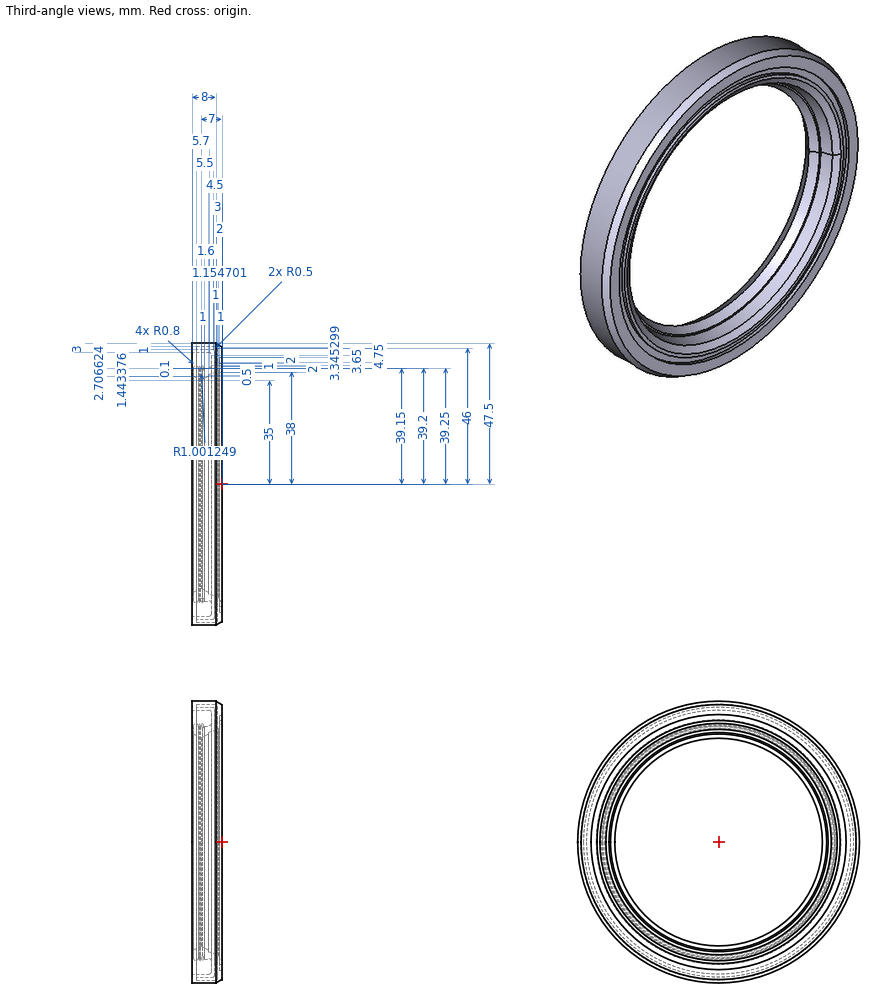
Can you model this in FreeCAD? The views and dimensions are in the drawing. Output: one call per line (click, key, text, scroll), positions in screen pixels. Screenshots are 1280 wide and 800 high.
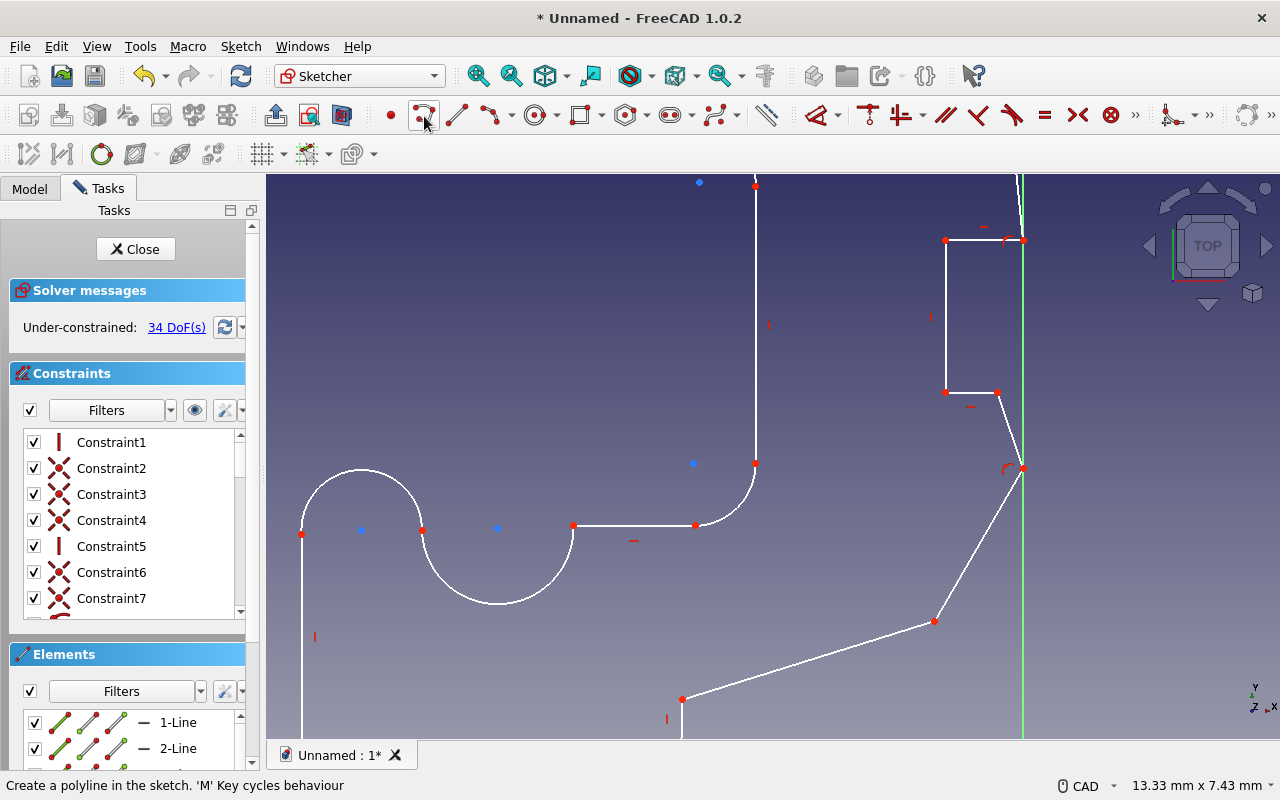
scroll(740, 507, down, 5)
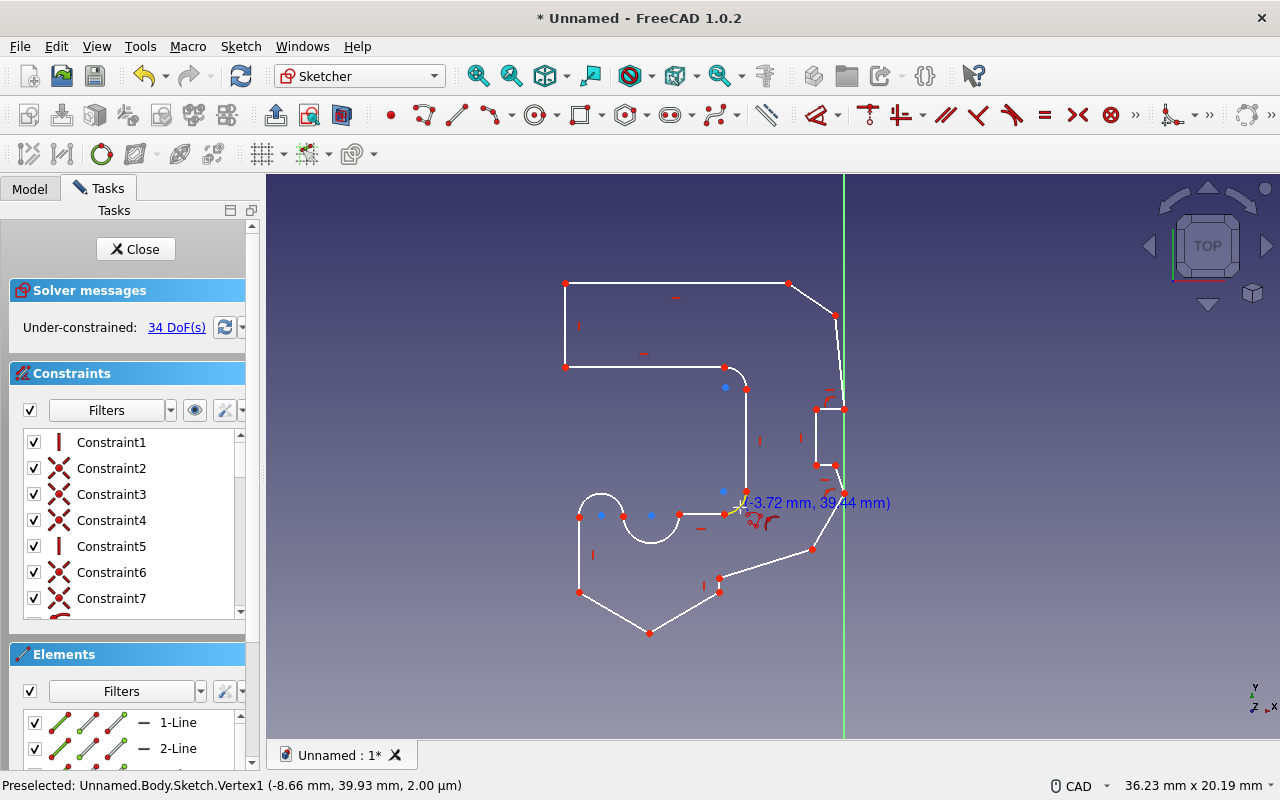
click(760, 338)
click(607, 338)
click(607, 310)
click(788, 310)
right_click(788, 310)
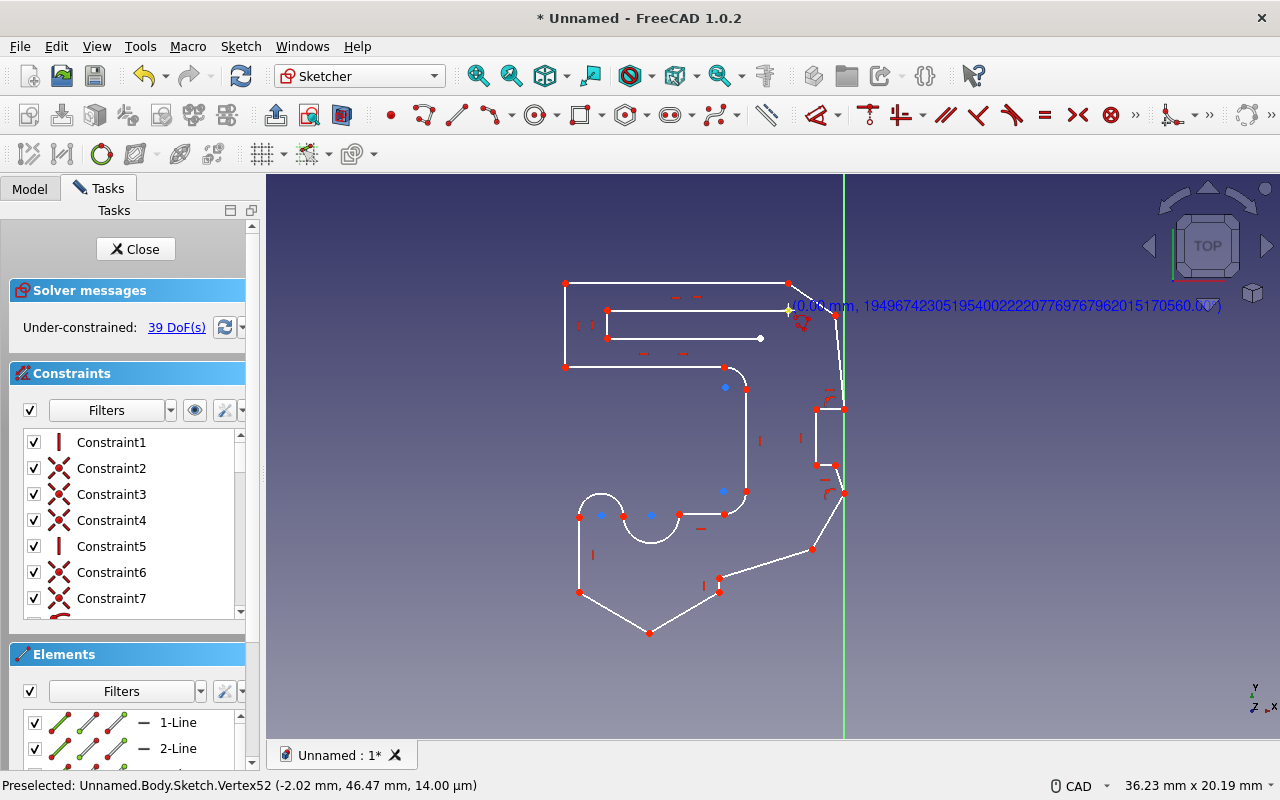
click(802, 324)
click(802, 457)
click(774, 457)
click(774, 352)
right_click(774, 352)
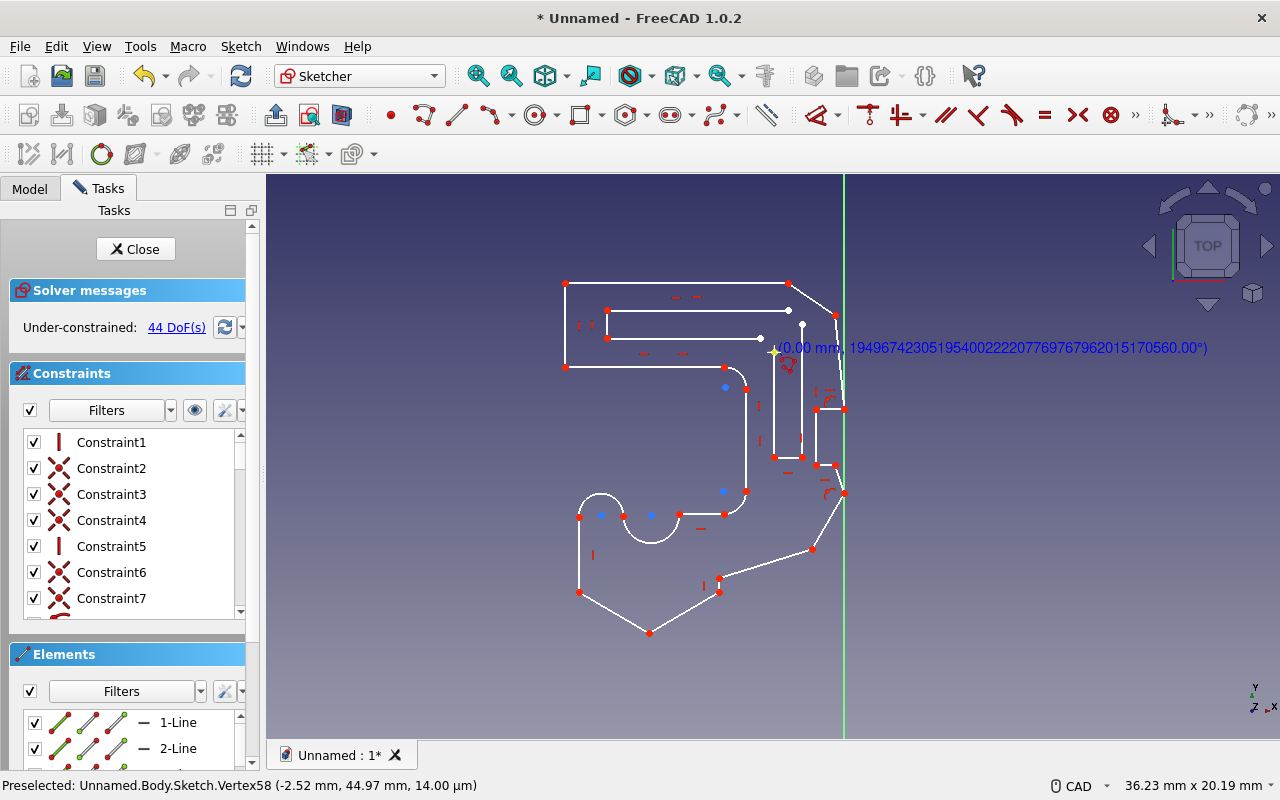
click(490, 116)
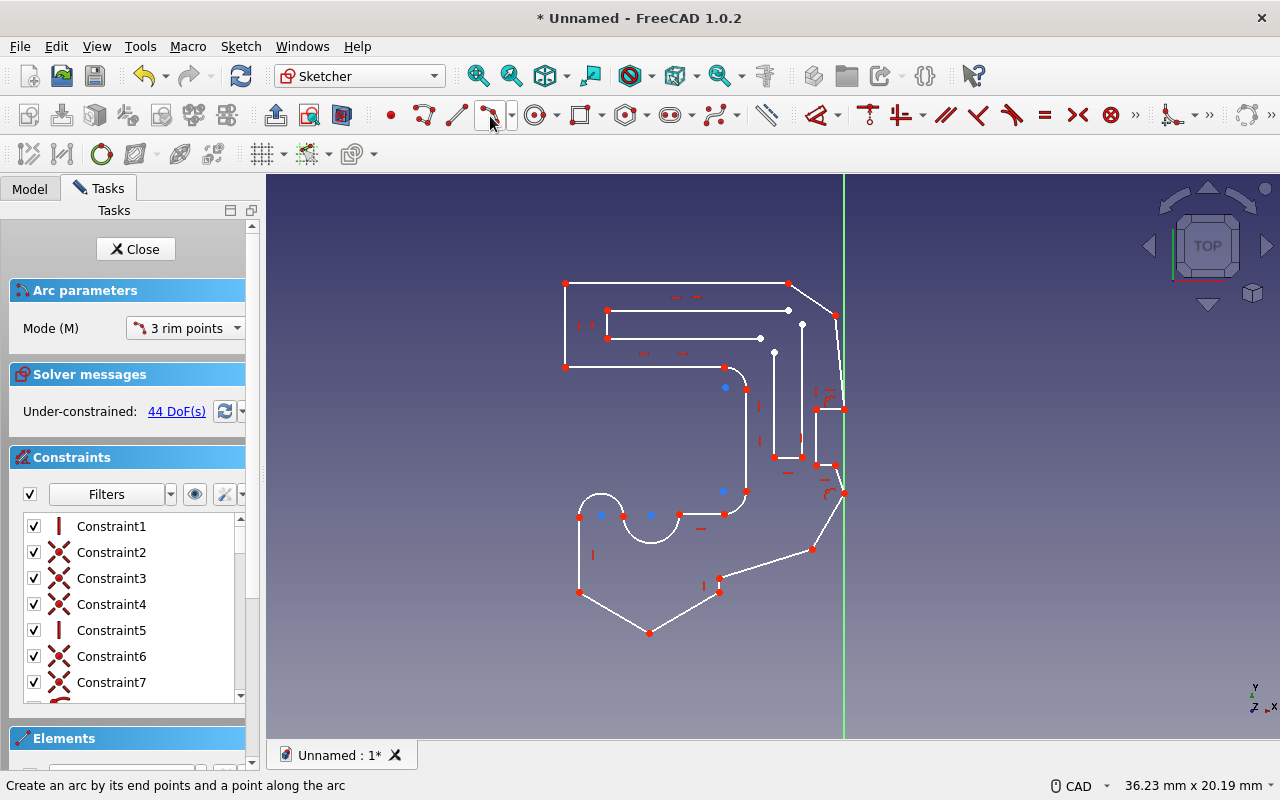
click(788, 311)
click(802, 325)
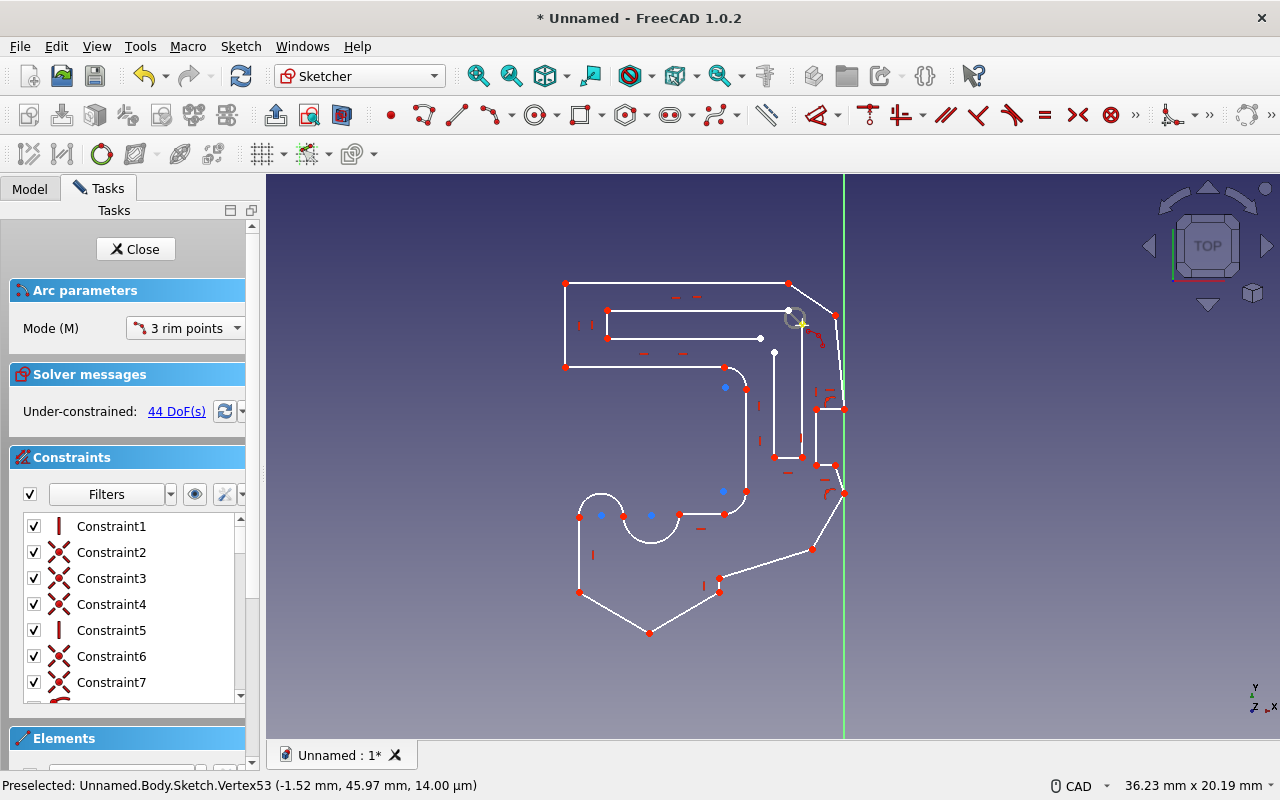
scroll(798, 314, up, 7)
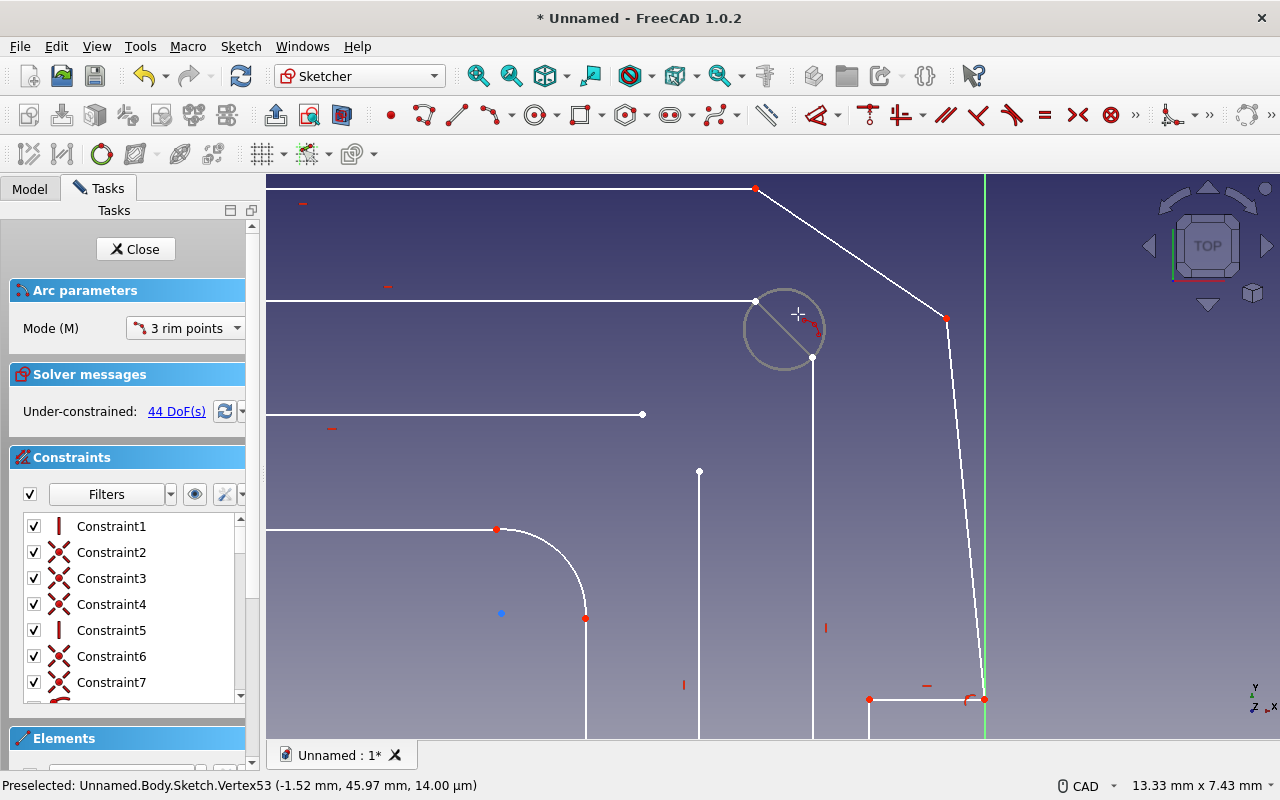
click(798, 315)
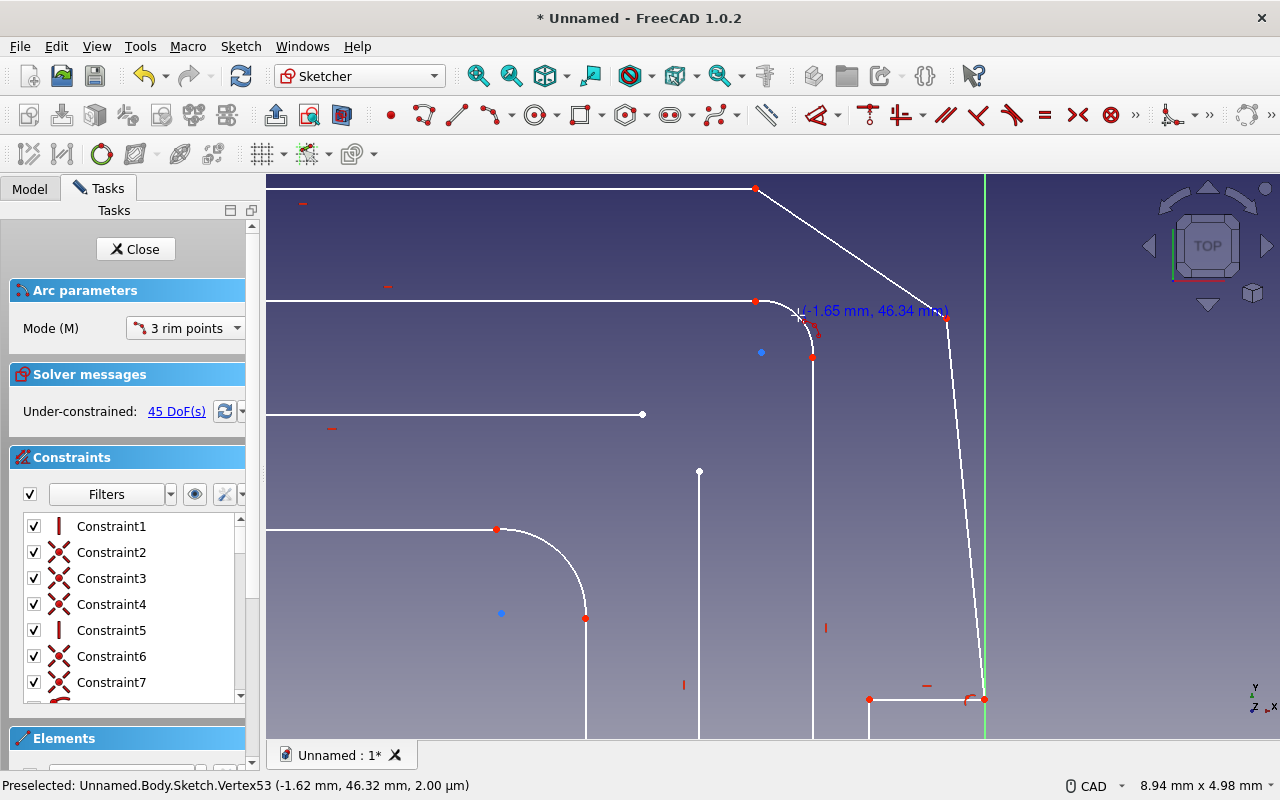
scroll(799, 313, down, 7)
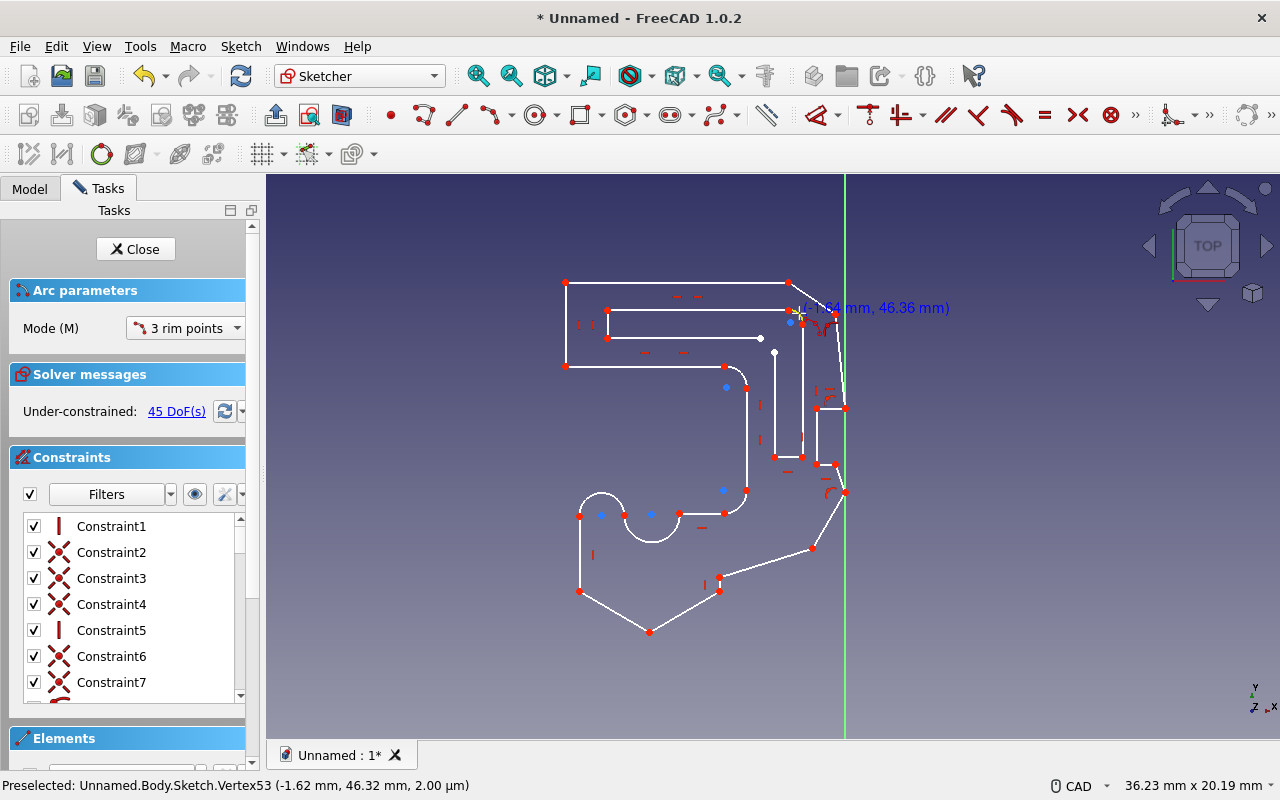
click(775, 352)
click(761, 338)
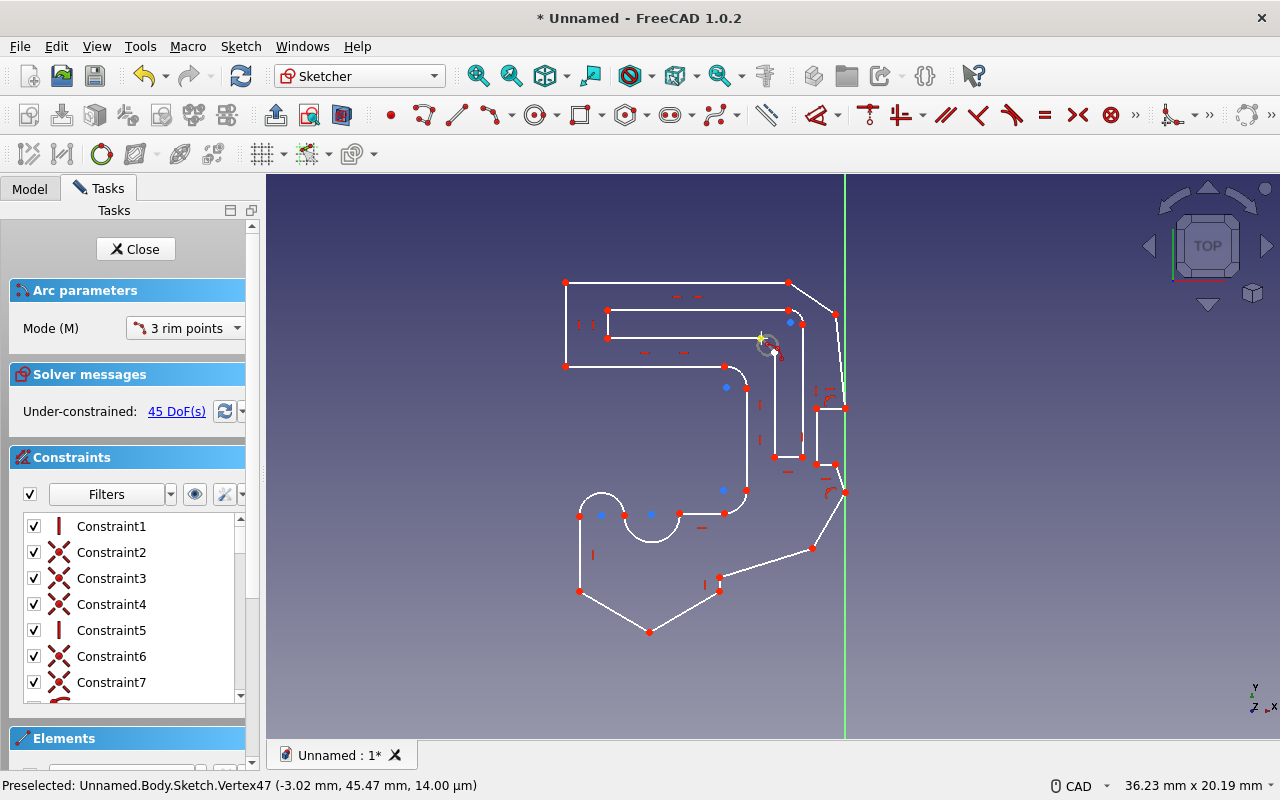
scroll(771, 342, up, 7)